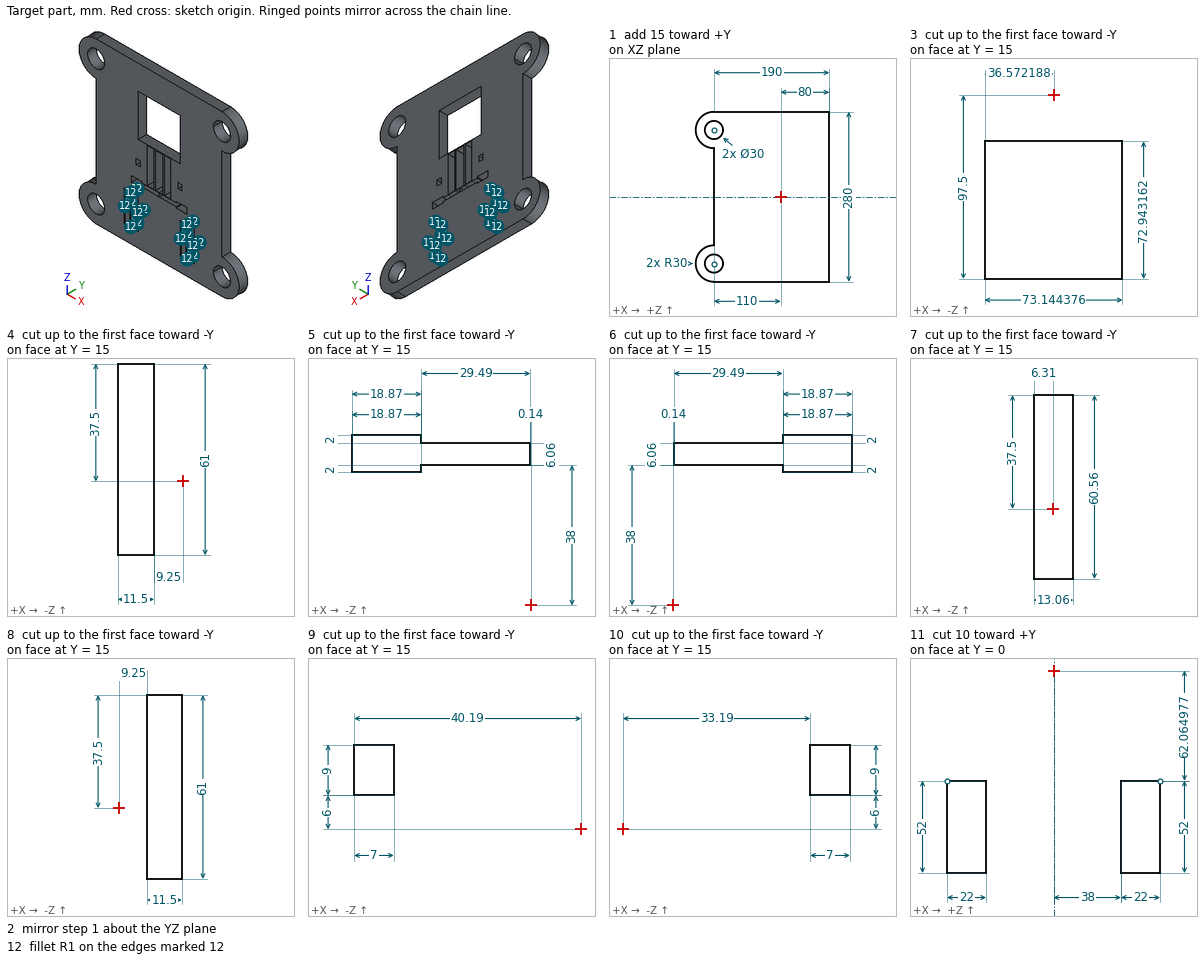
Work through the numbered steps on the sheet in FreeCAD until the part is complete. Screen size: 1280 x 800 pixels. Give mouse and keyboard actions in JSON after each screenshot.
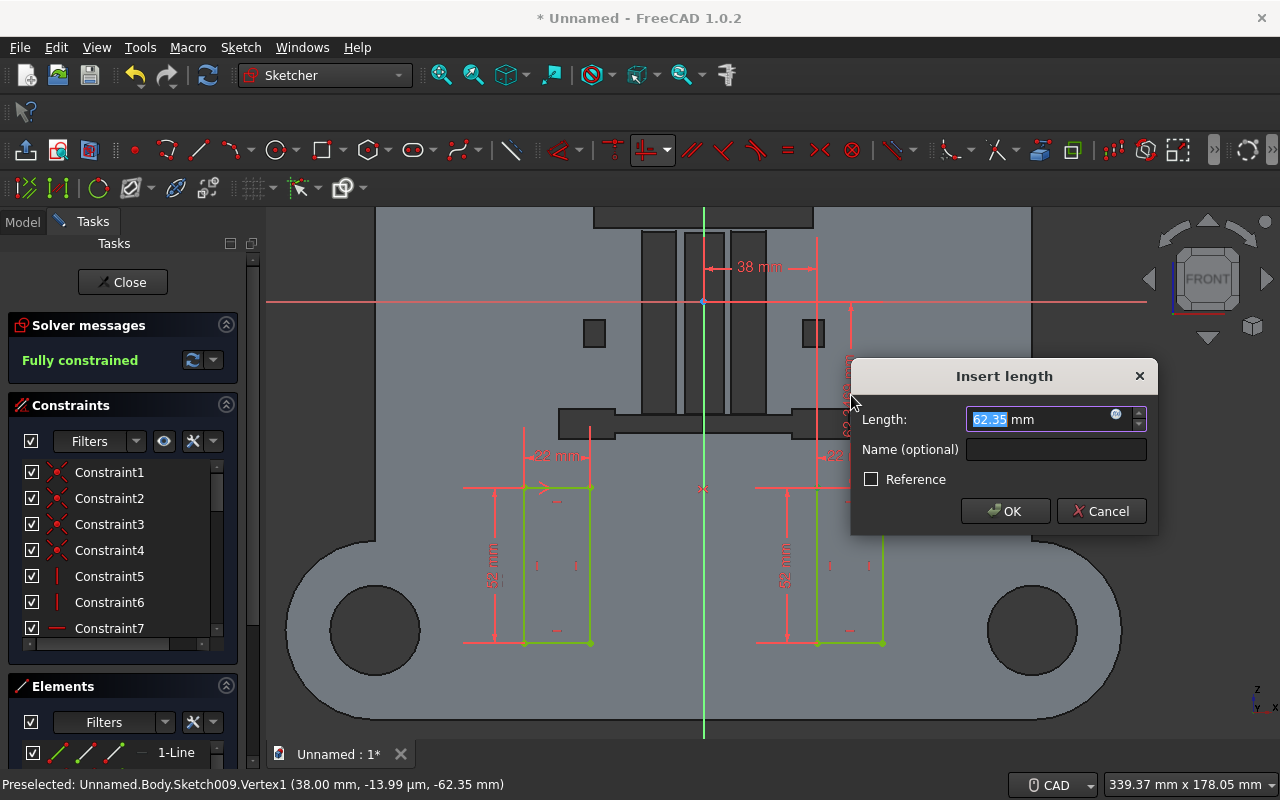
{"action": "type", "text": "62.064977"}
{"action": "key", "text": "Return"}
{"action": "key", "text": "Escape"}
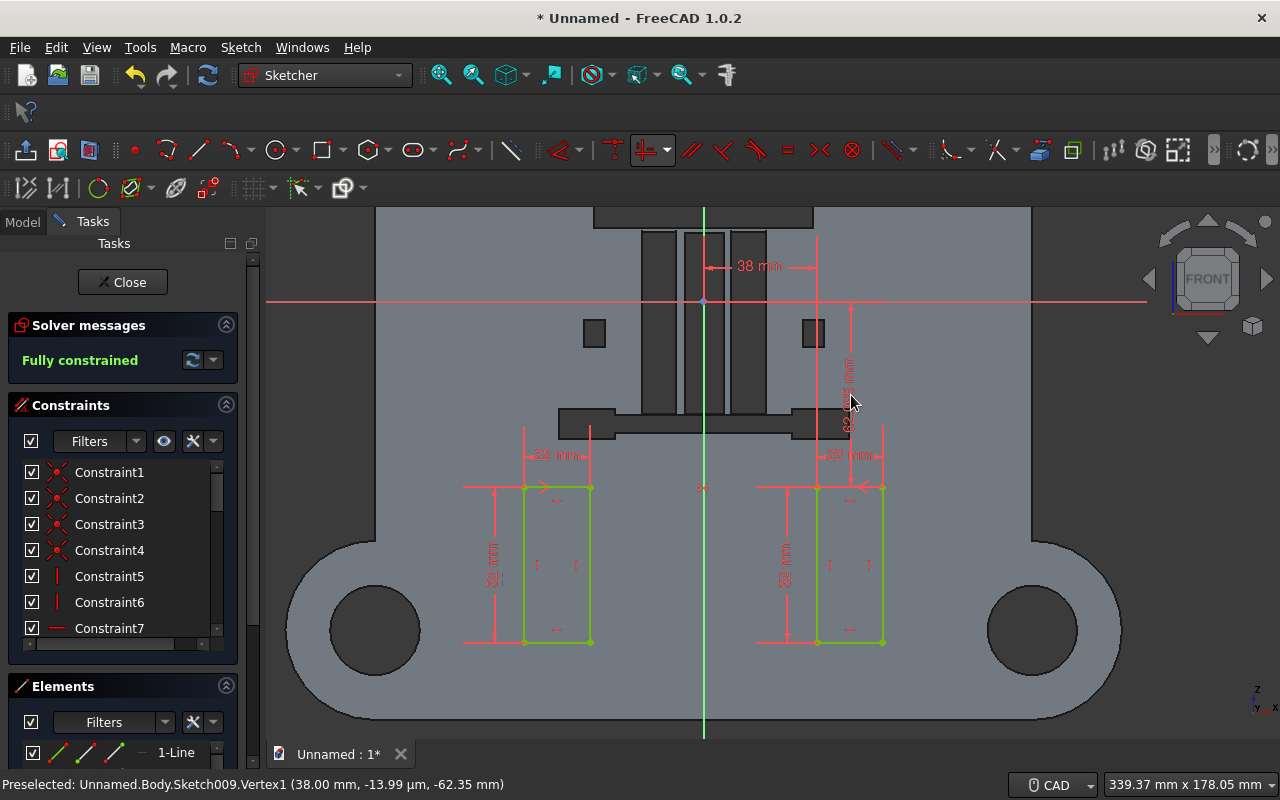
{"action": "left_click", "coordinate": [123, 282]}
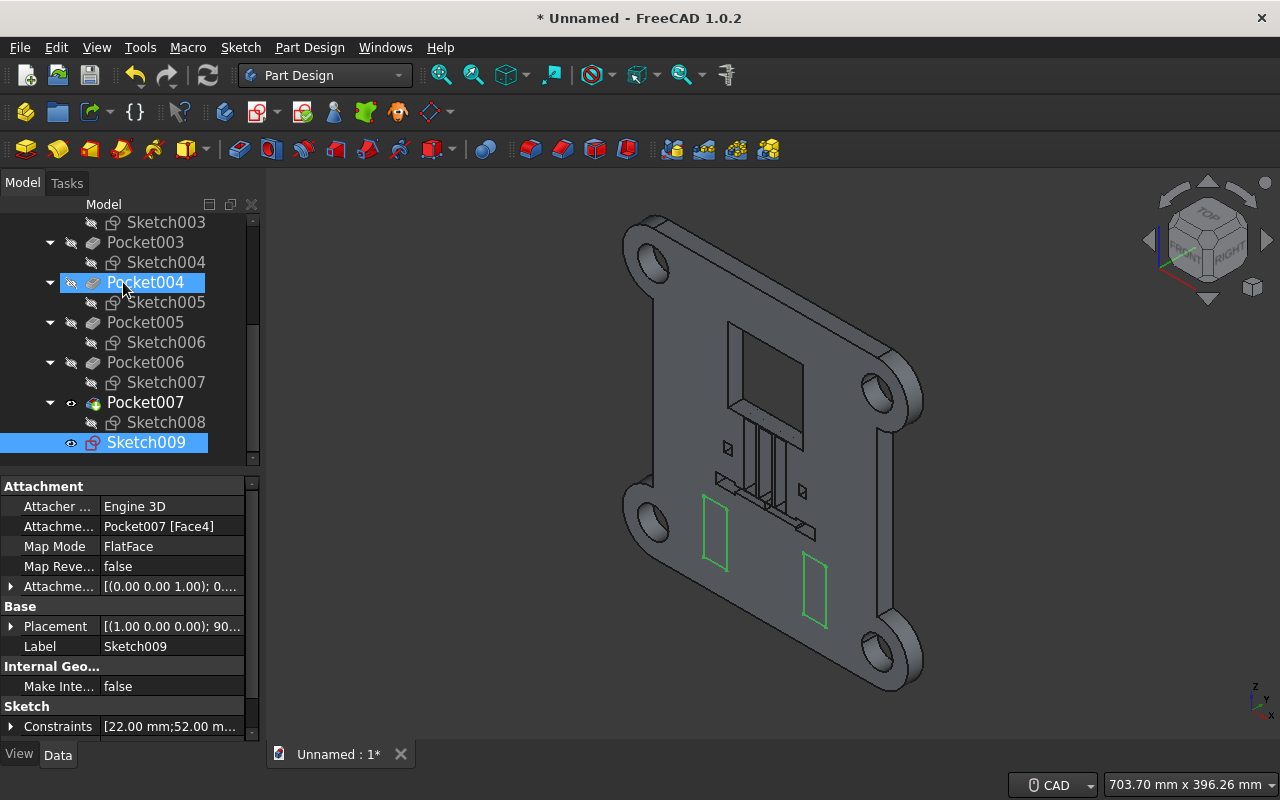
{"action": "left_click", "coordinate": [240, 150]}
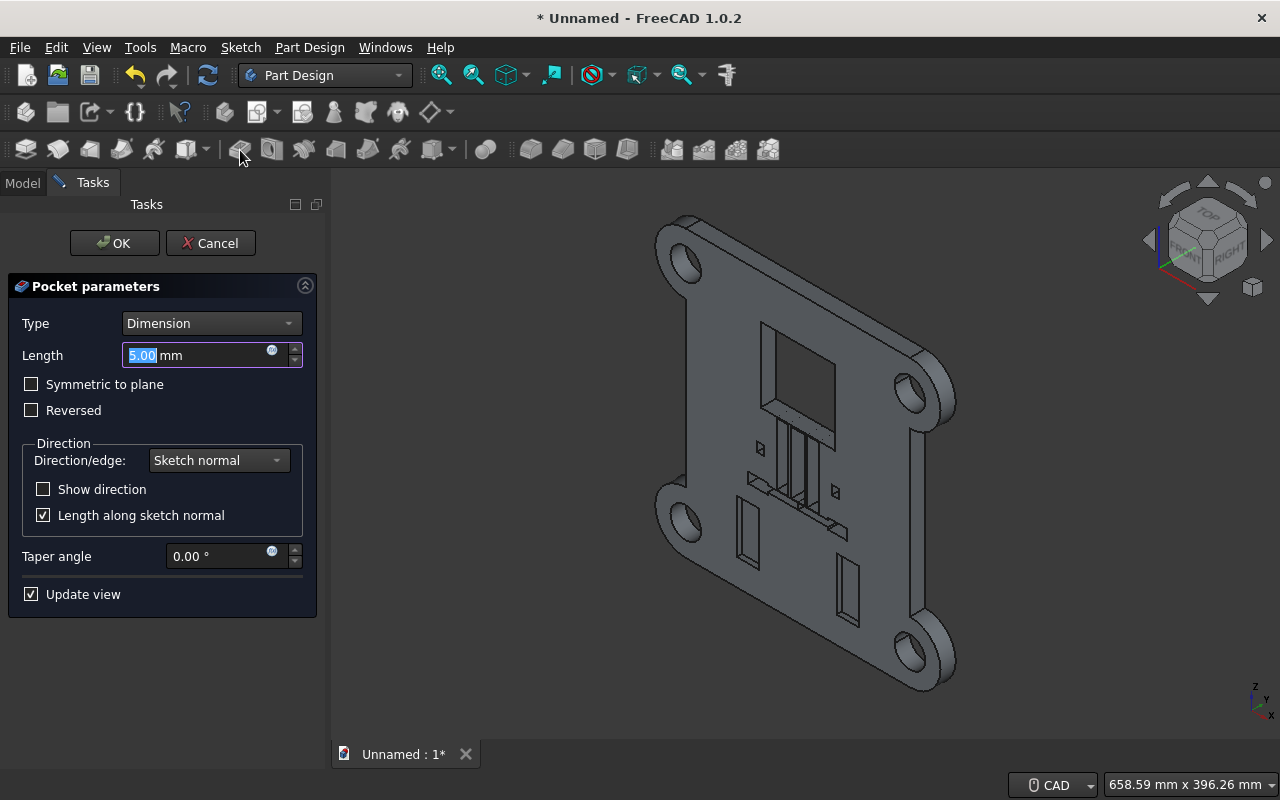
{"action": "type", "text": "10"}
{"action": "key", "text": "Tab"}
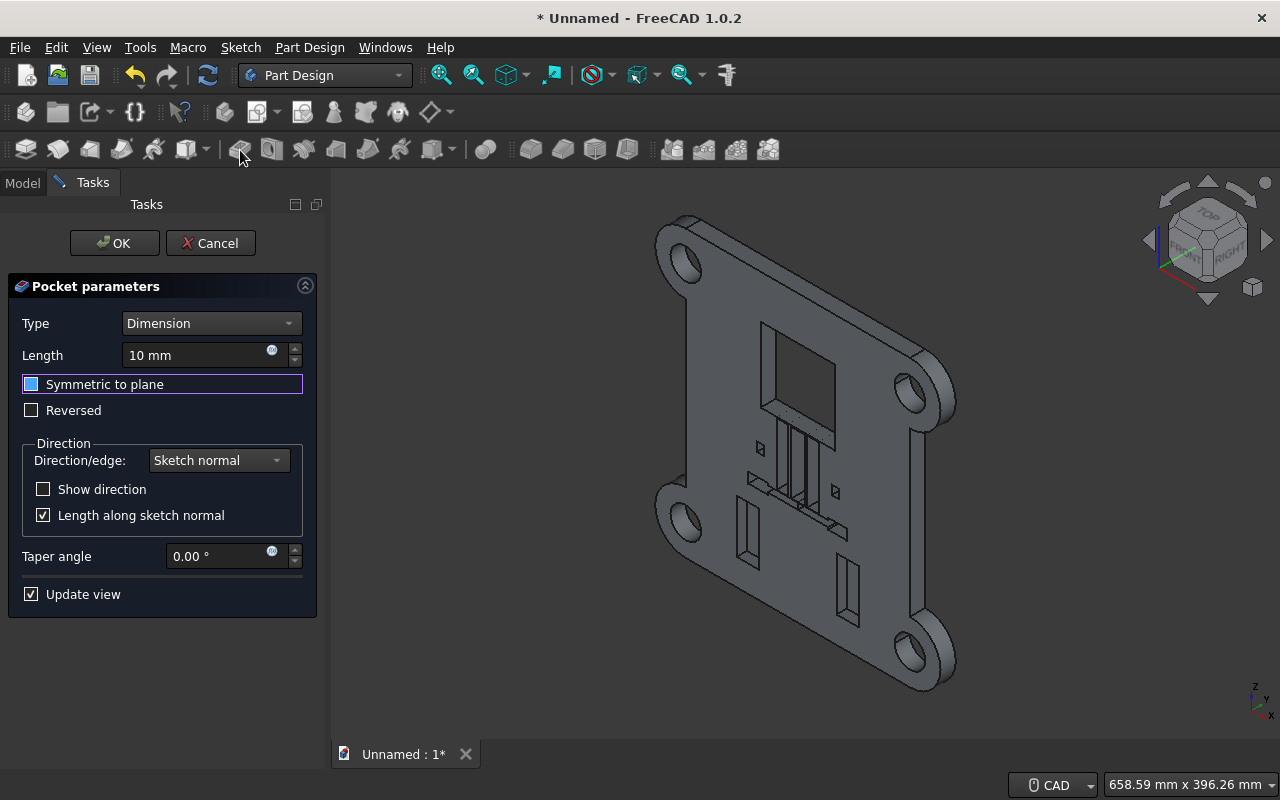
{"action": "left_click", "coordinate": [115, 243]}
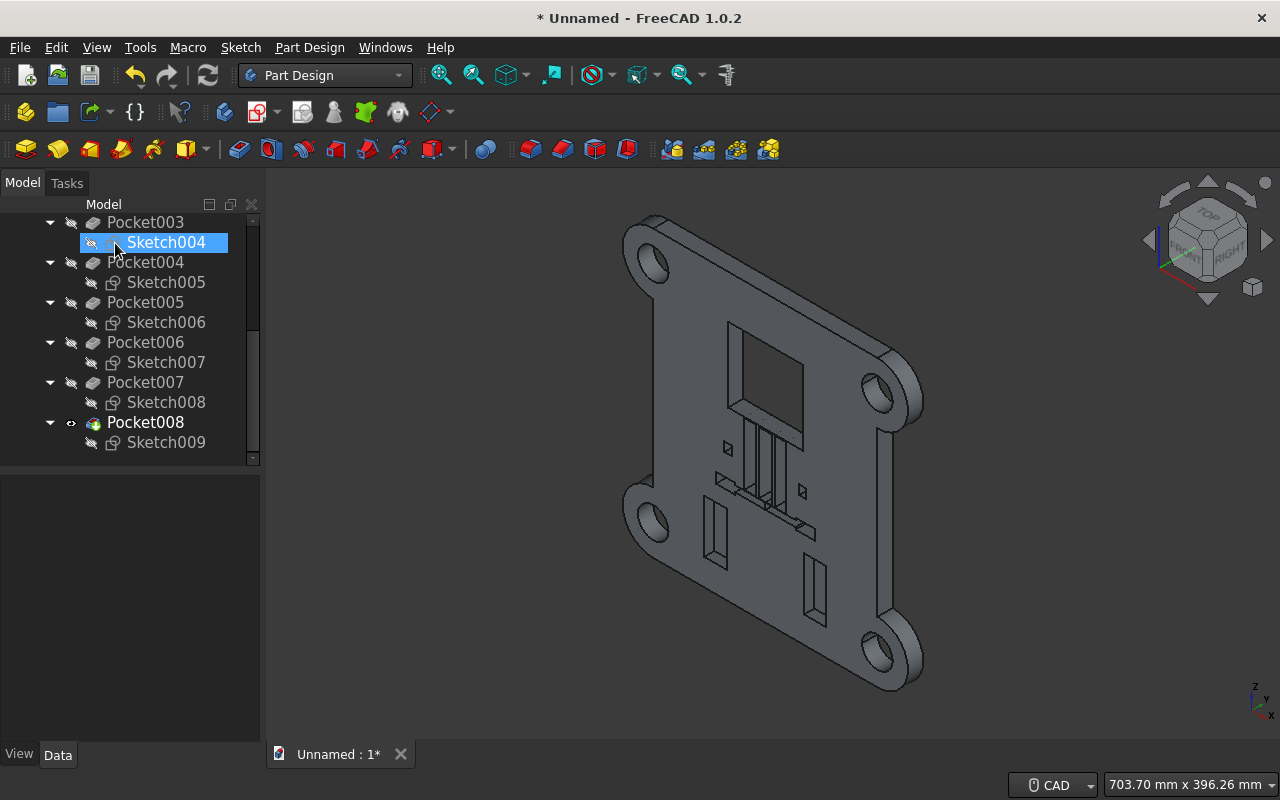
{"action": "left_click", "coordinate": [804, 583]}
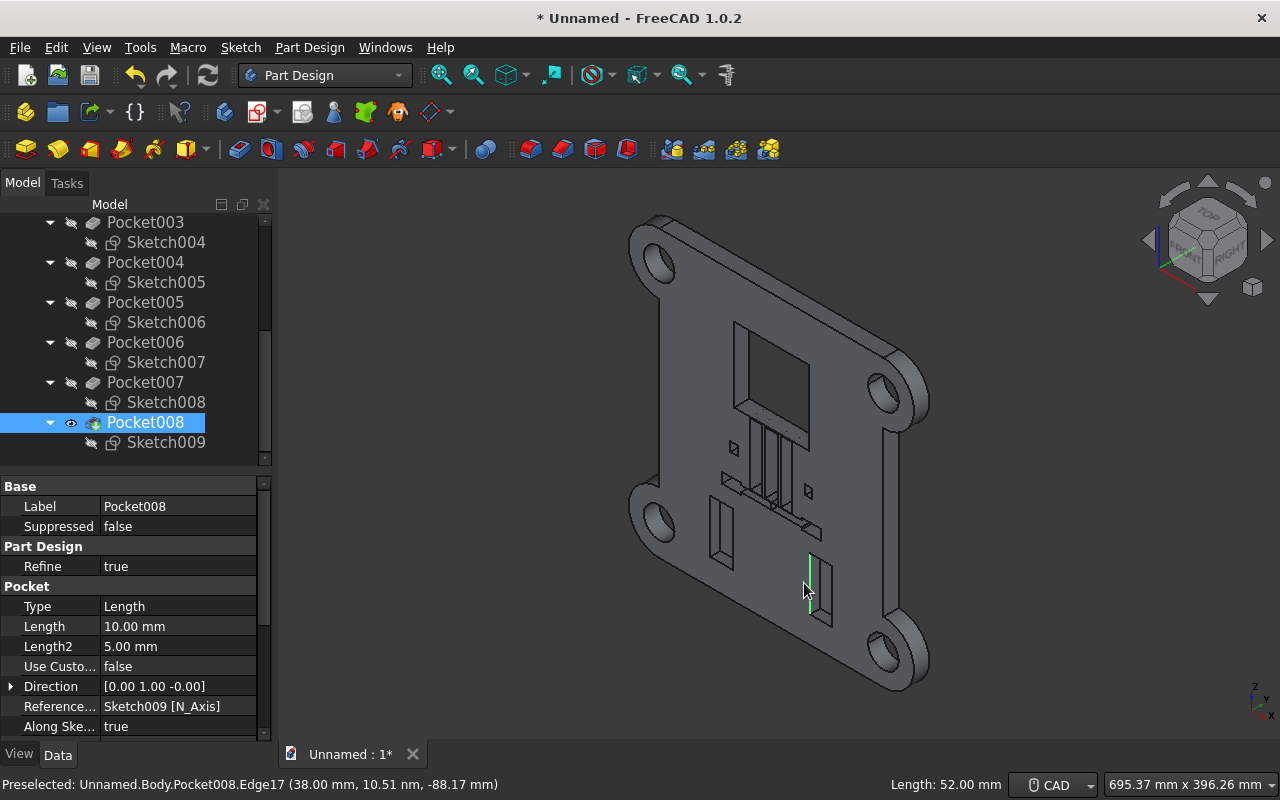
{"action": "left_click", "coordinate": [821, 620], "text": "ctrl"}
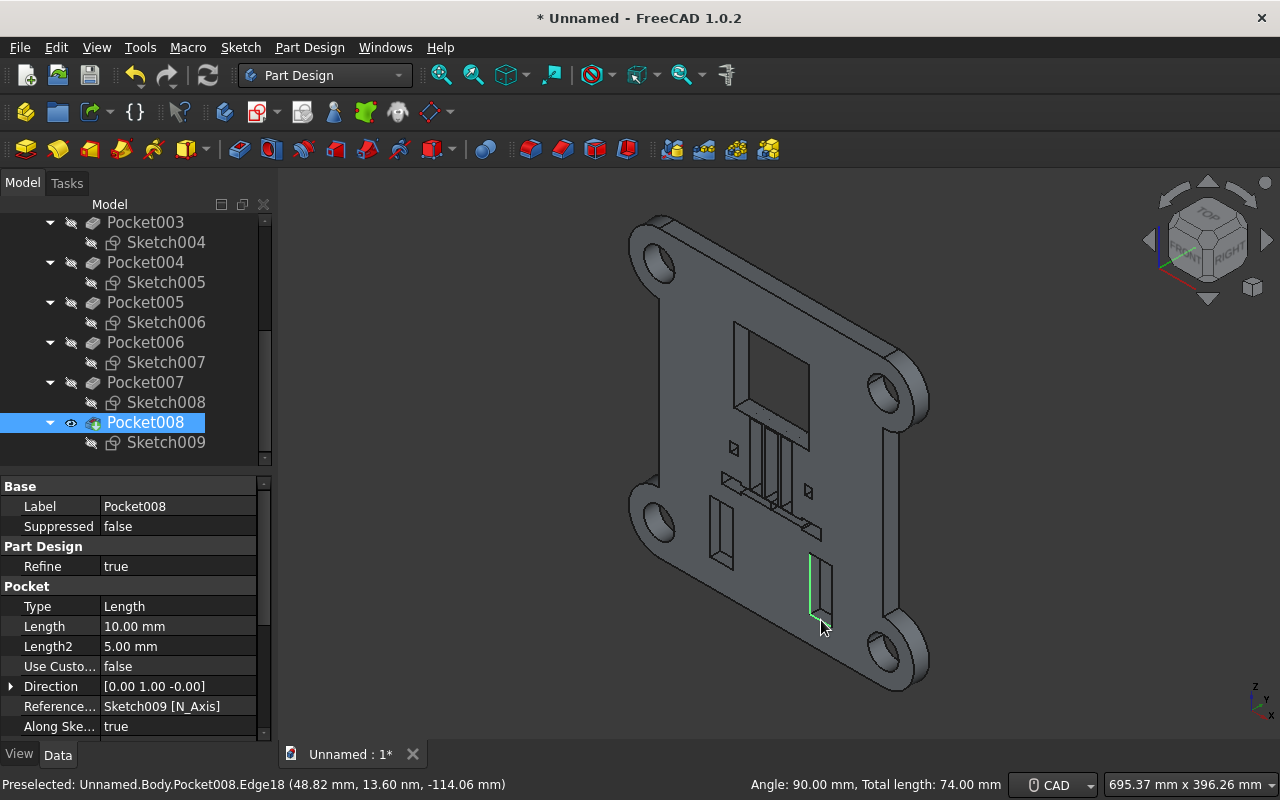
{"action": "left_click", "coordinate": [710, 525], "text": "ctrl"}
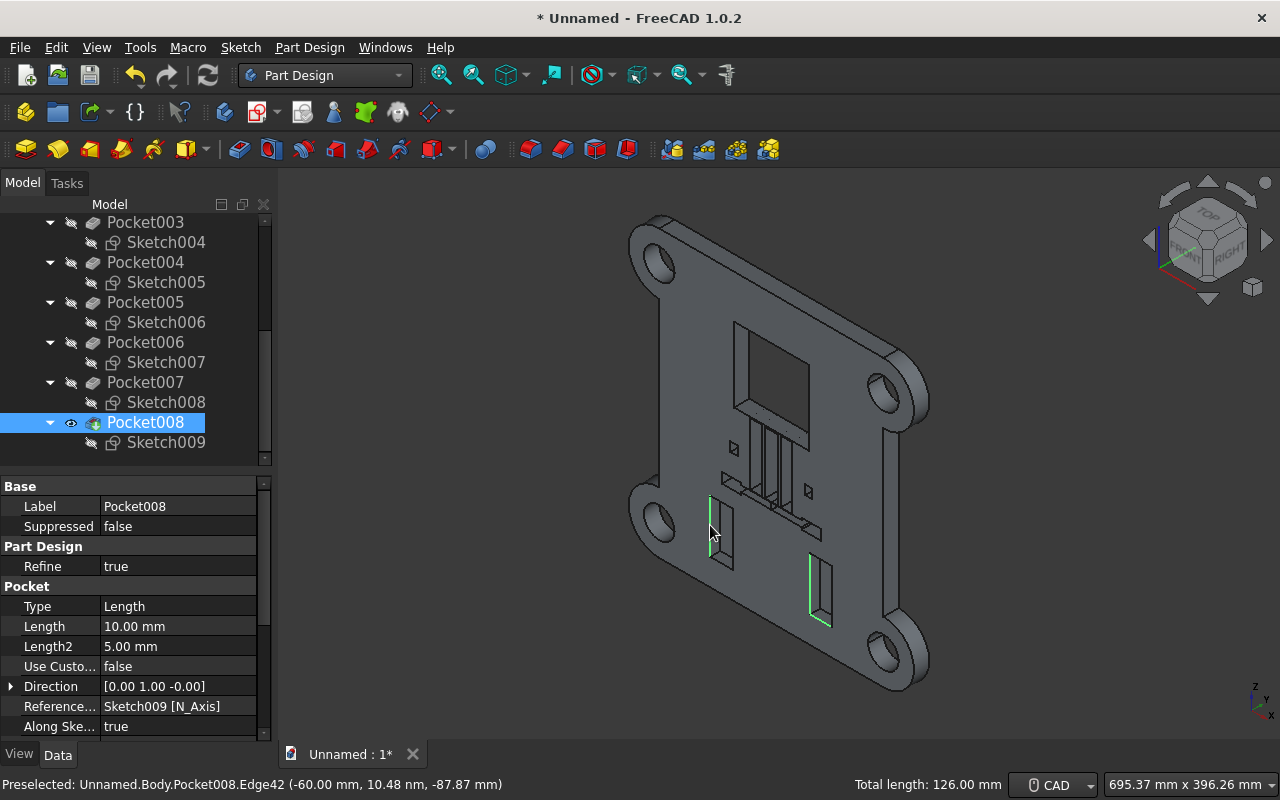
{"action": "left_click", "coordinate": [721, 562], "text": "ctrl"}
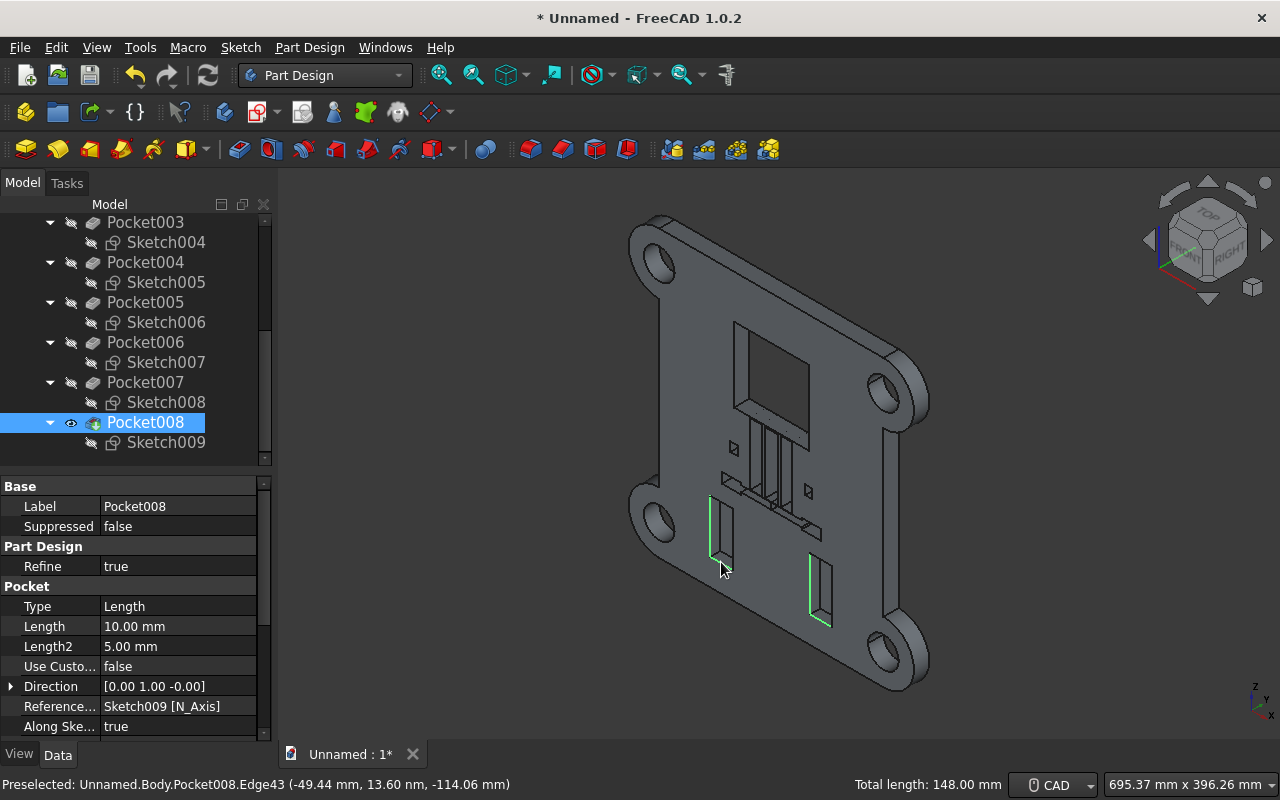
{"action": "key", "text": "2"}